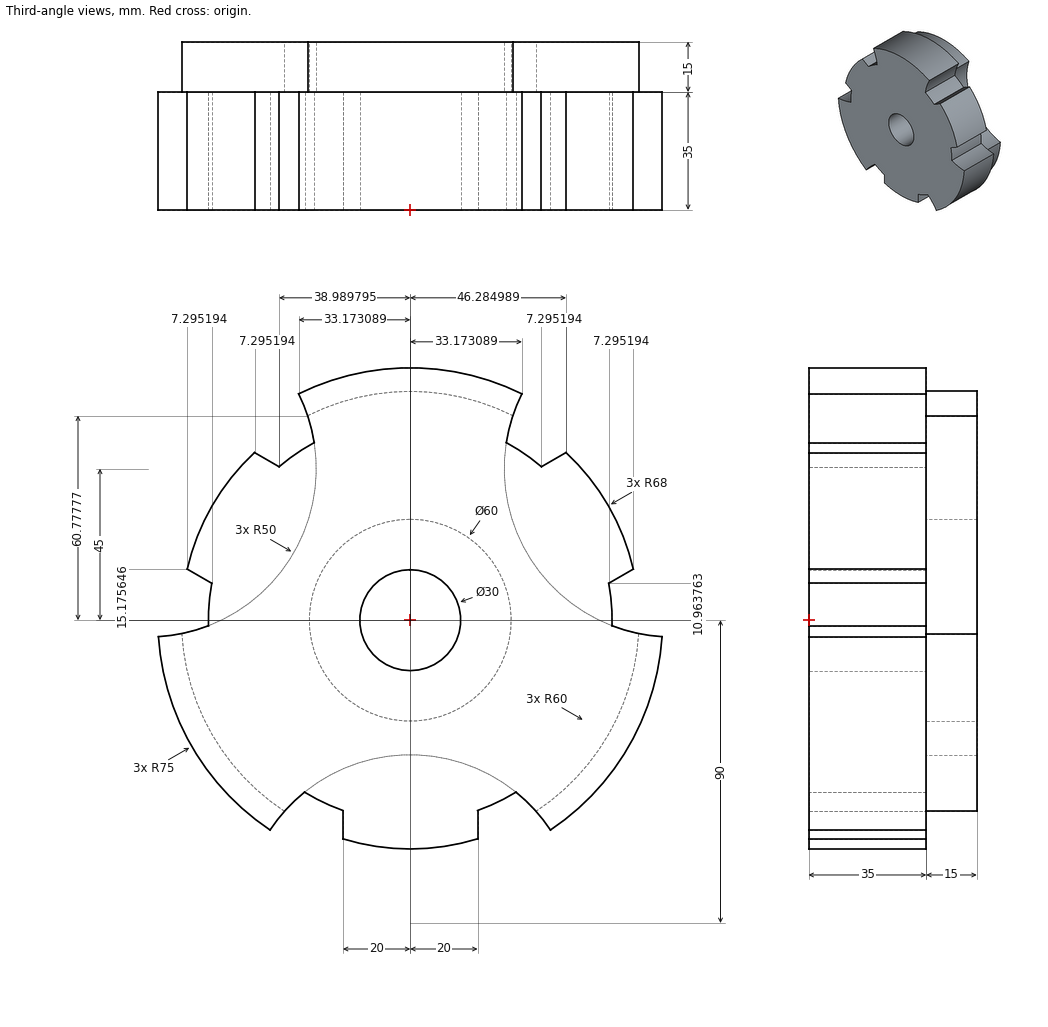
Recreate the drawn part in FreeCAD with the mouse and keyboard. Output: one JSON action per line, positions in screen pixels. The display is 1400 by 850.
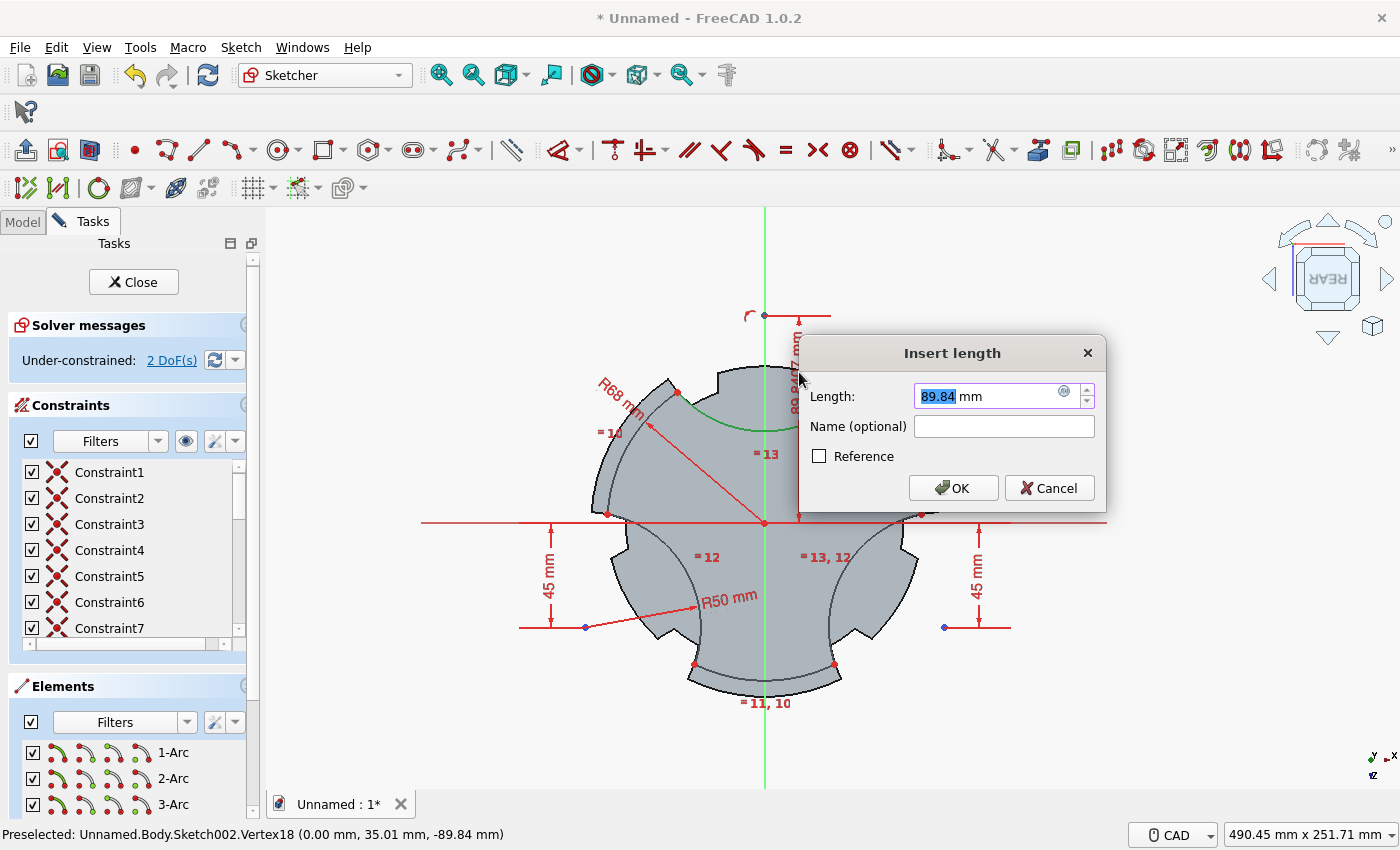
{"action": "type", "text": "90"}
{"action": "key", "text": "Return"}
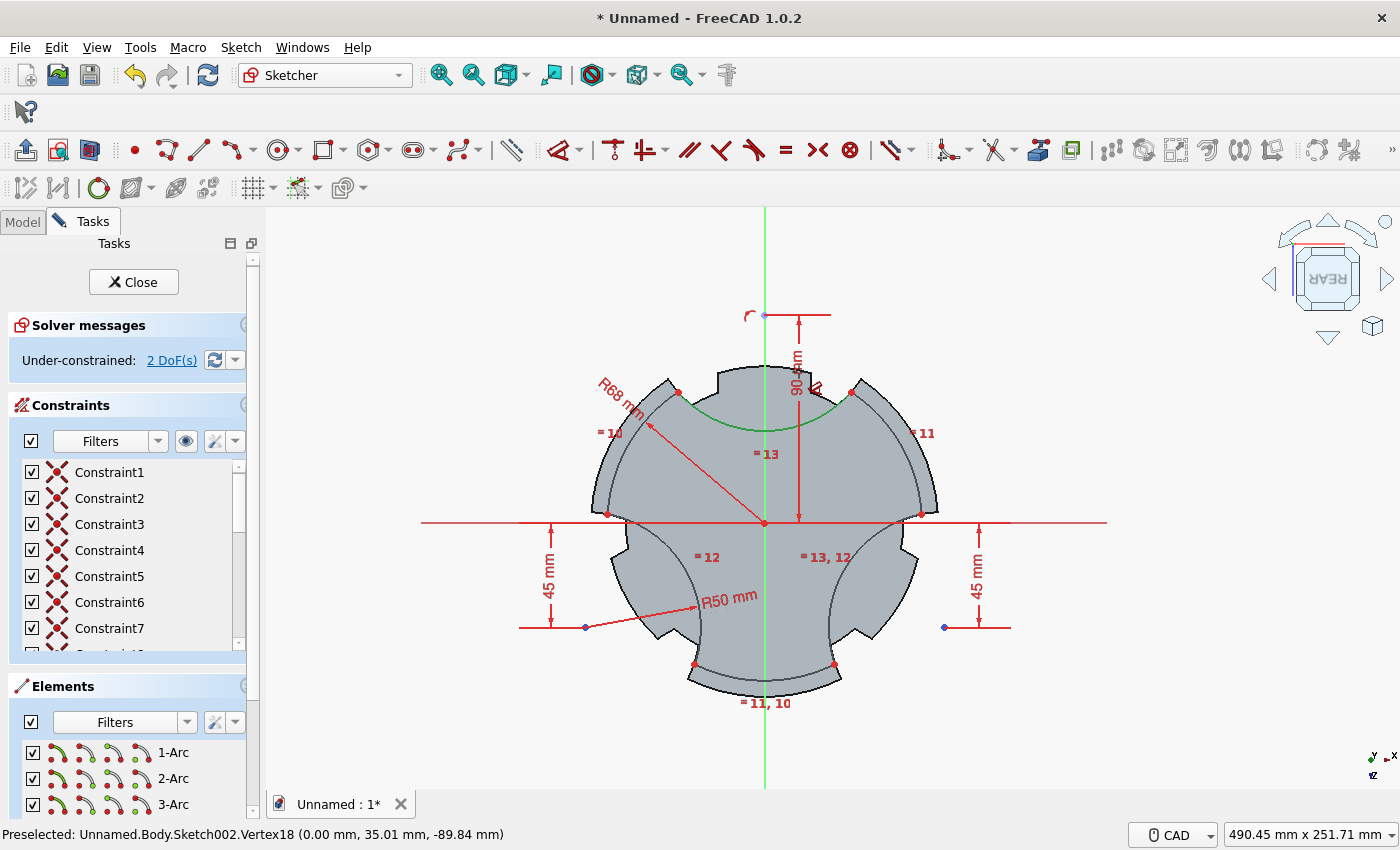
{"action": "left_click", "coordinate": [695, 664]}
{"action": "left_click", "coordinate": [661, 561]}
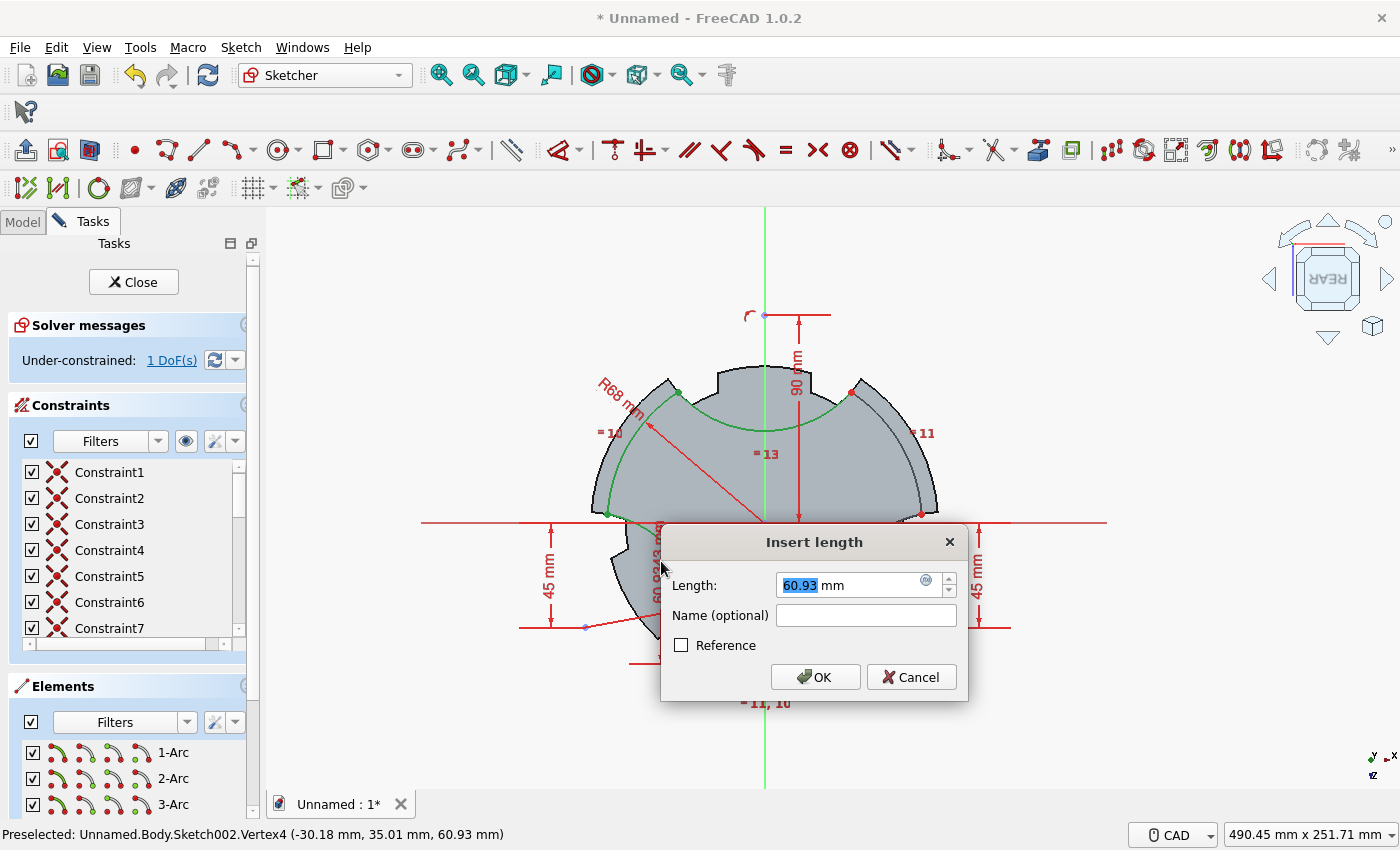
{"action": "type", "text": "60.77777"}
{"action": "key", "text": "Return"}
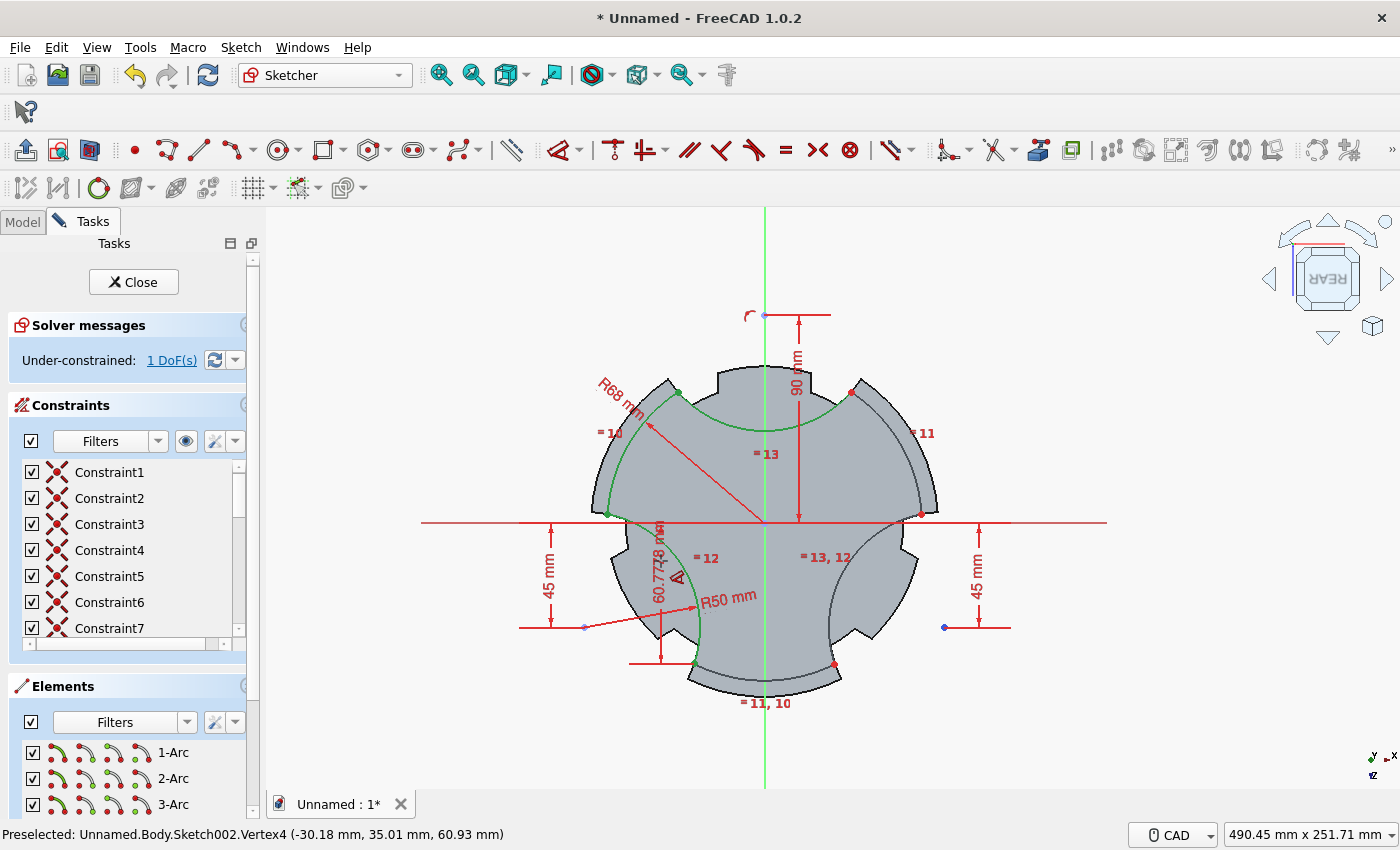
{"action": "left_click", "coordinate": [835, 664]}
{"action": "left_click", "coordinate": [869, 594]}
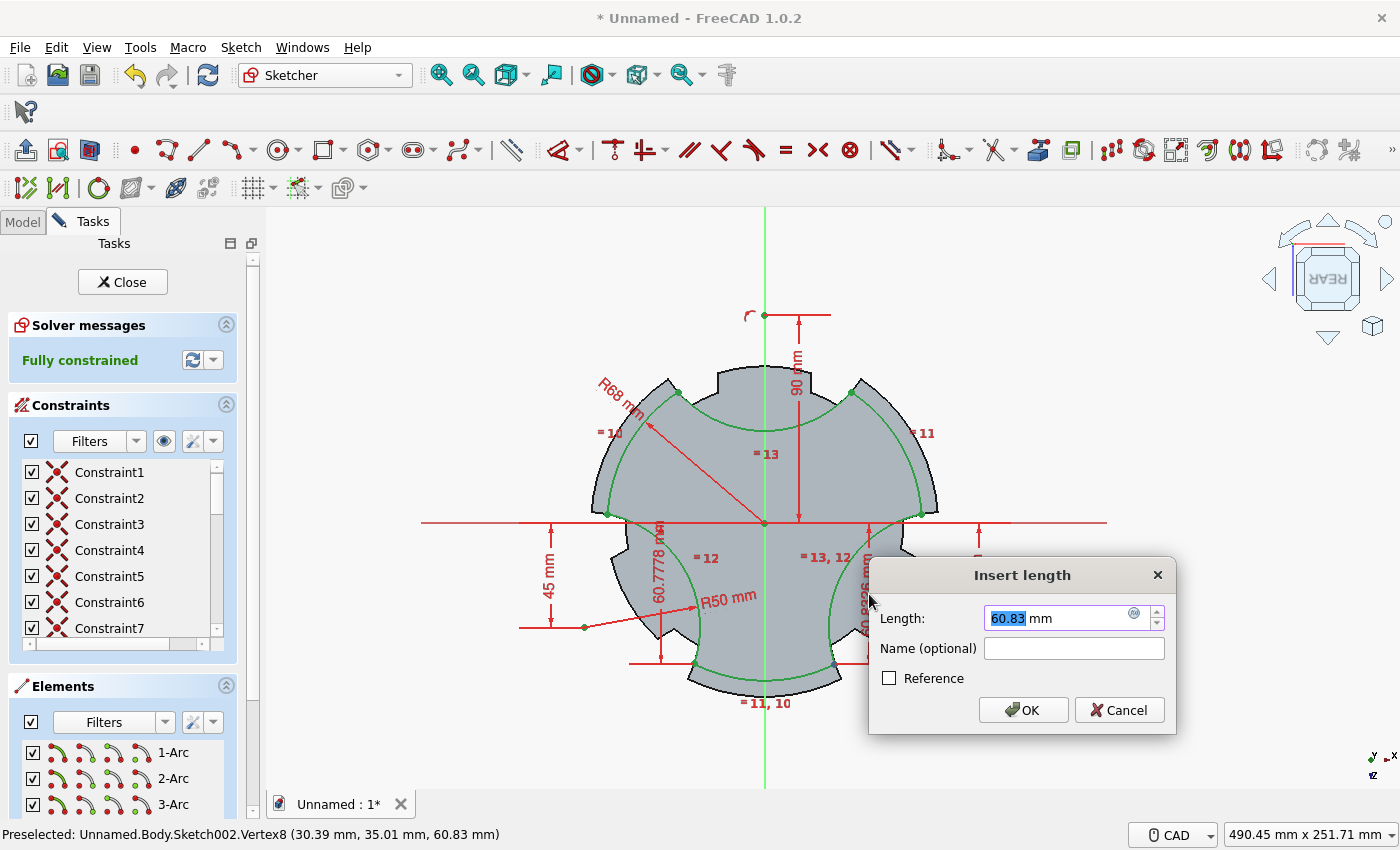
{"action": "type", "text": "60.77777"}
{"action": "key", "text": "Return"}
{"action": "key", "text": "Escape"}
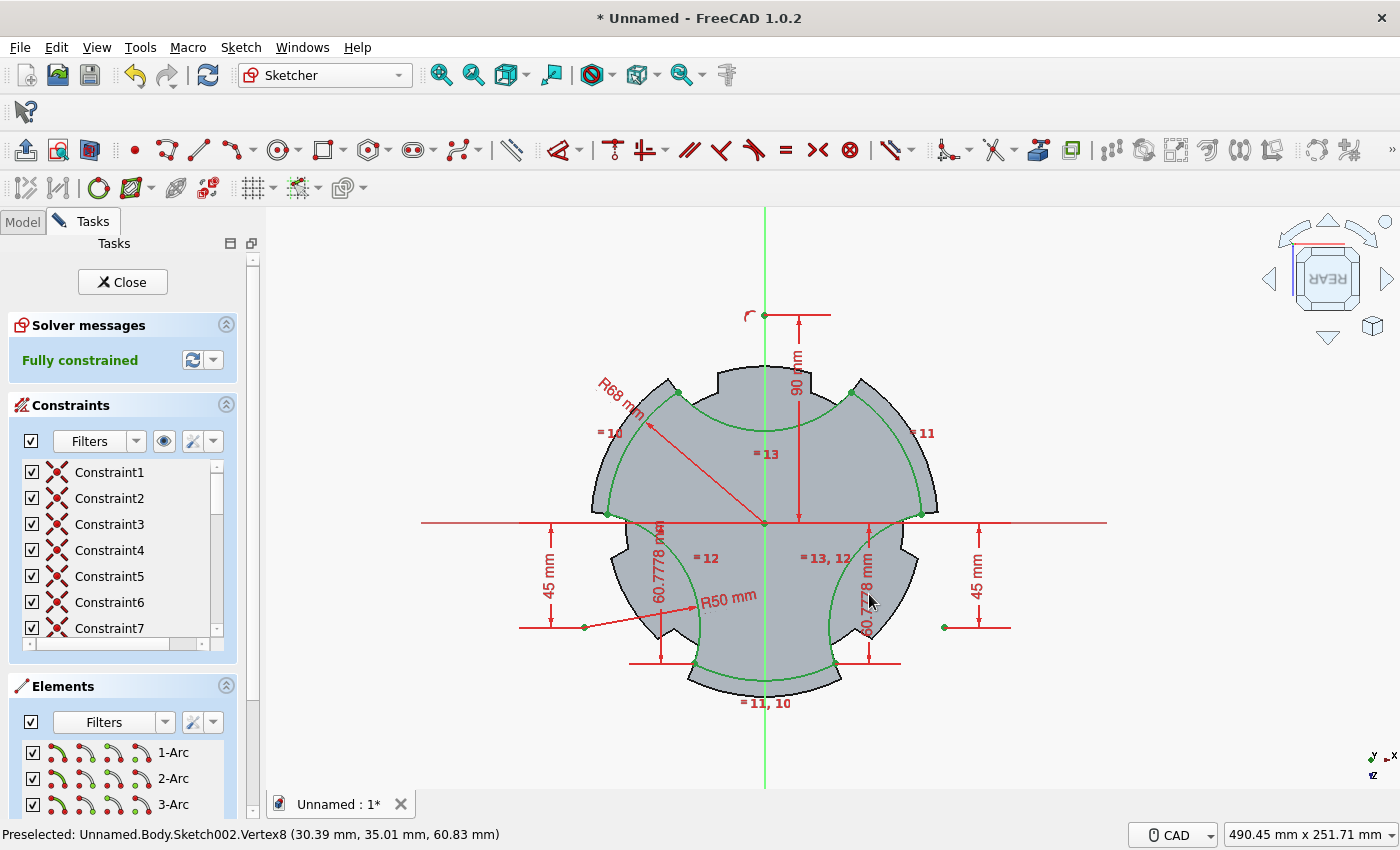
{"action": "left_click", "coordinate": [123, 282]}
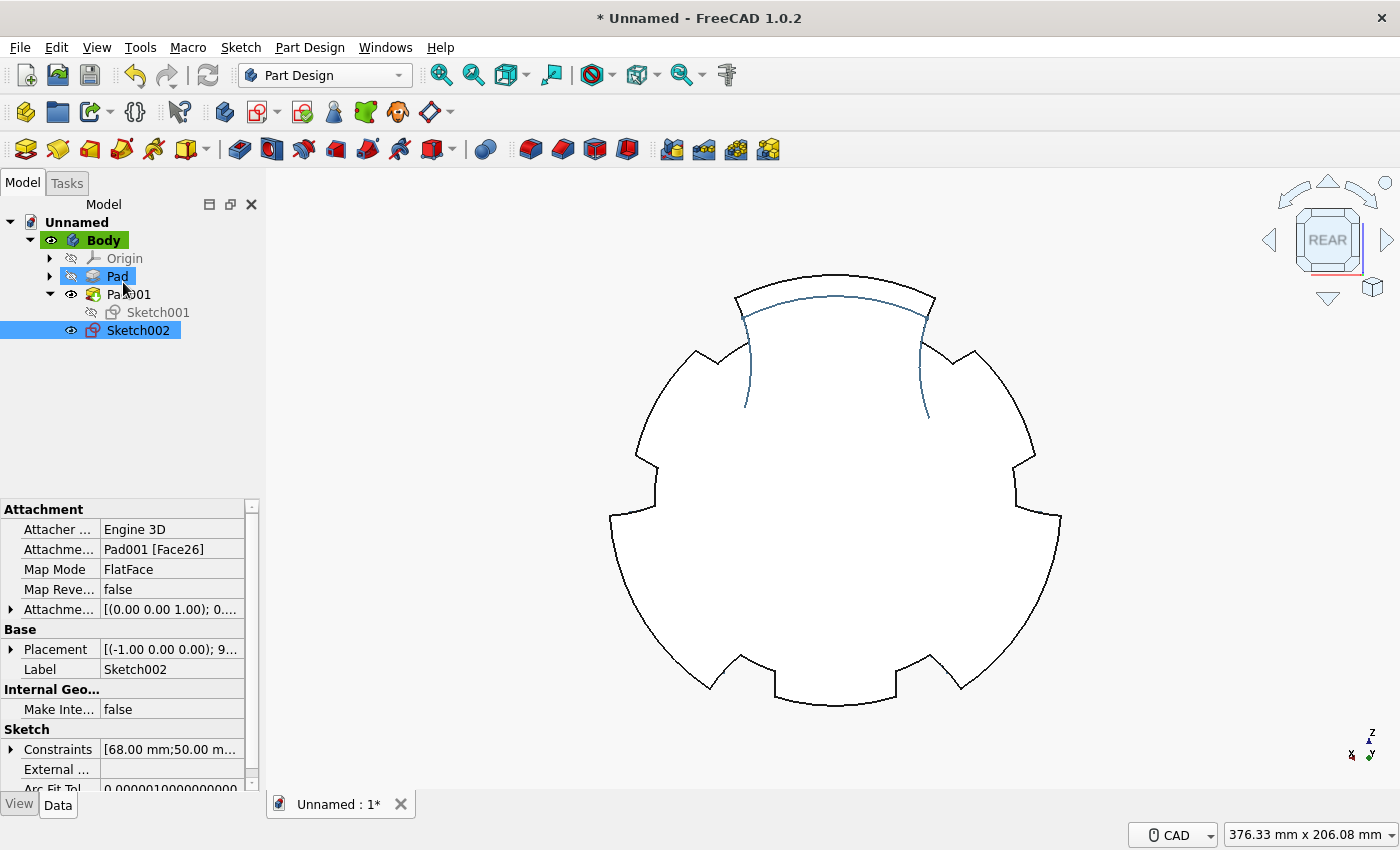
{"action": "left_click", "coordinate": [26, 150]}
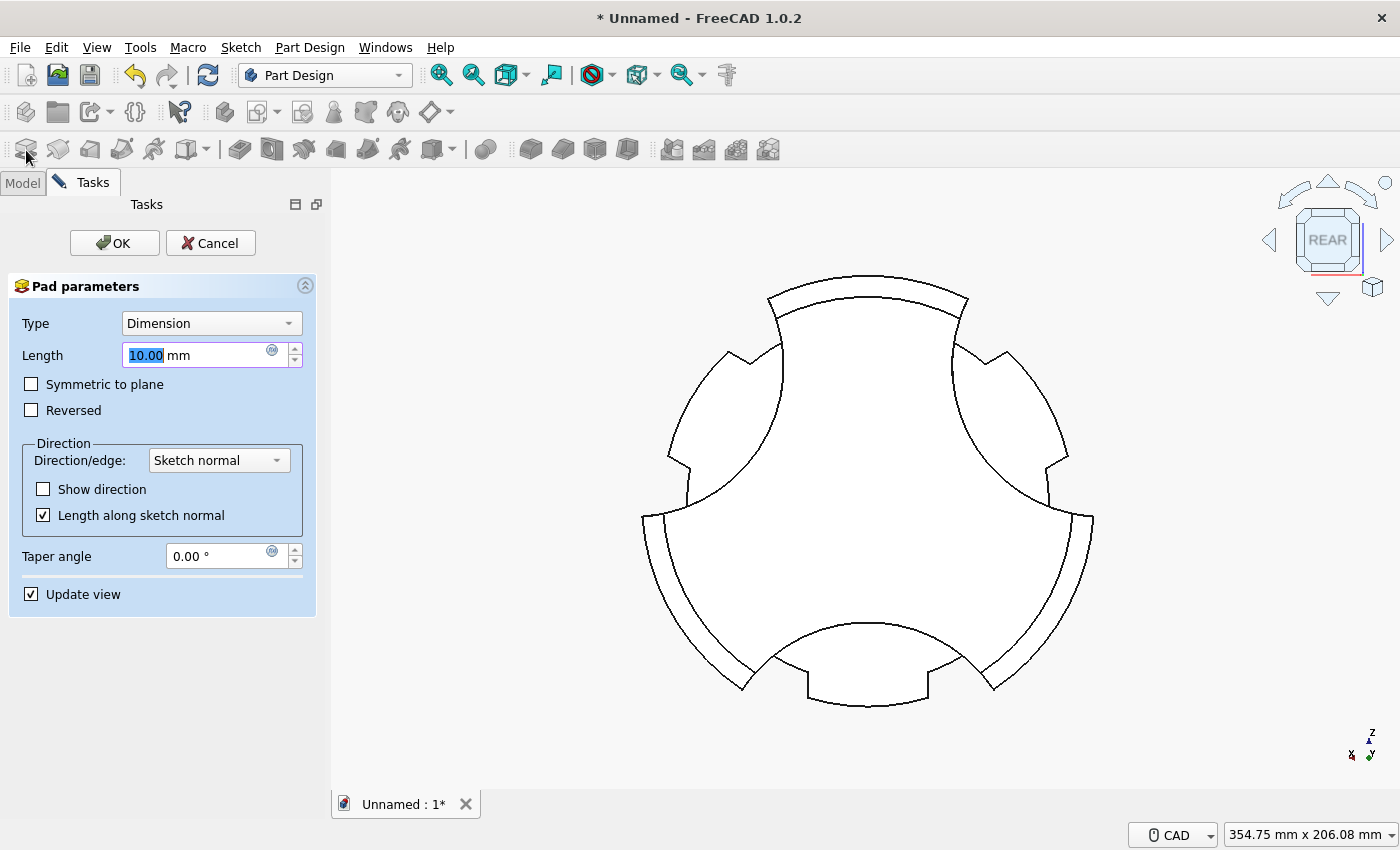
{"action": "type", "text": "15"}
{"action": "key", "text": "Tab"}